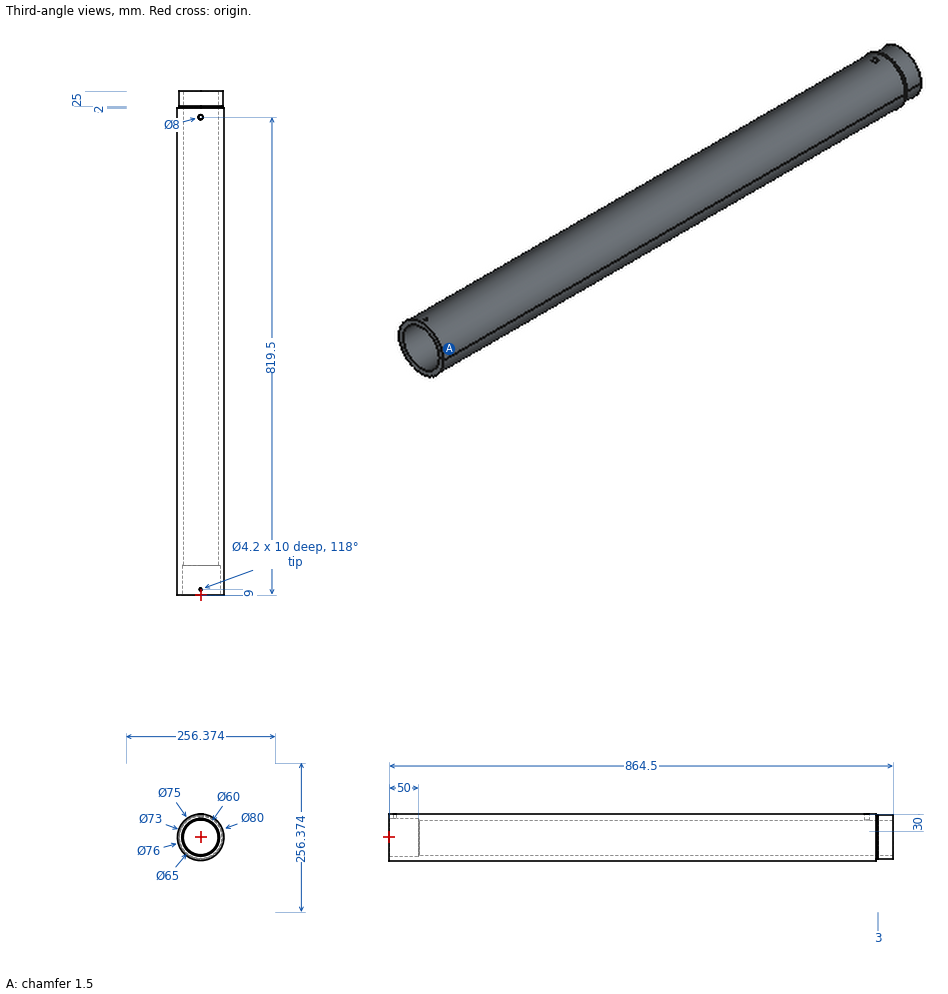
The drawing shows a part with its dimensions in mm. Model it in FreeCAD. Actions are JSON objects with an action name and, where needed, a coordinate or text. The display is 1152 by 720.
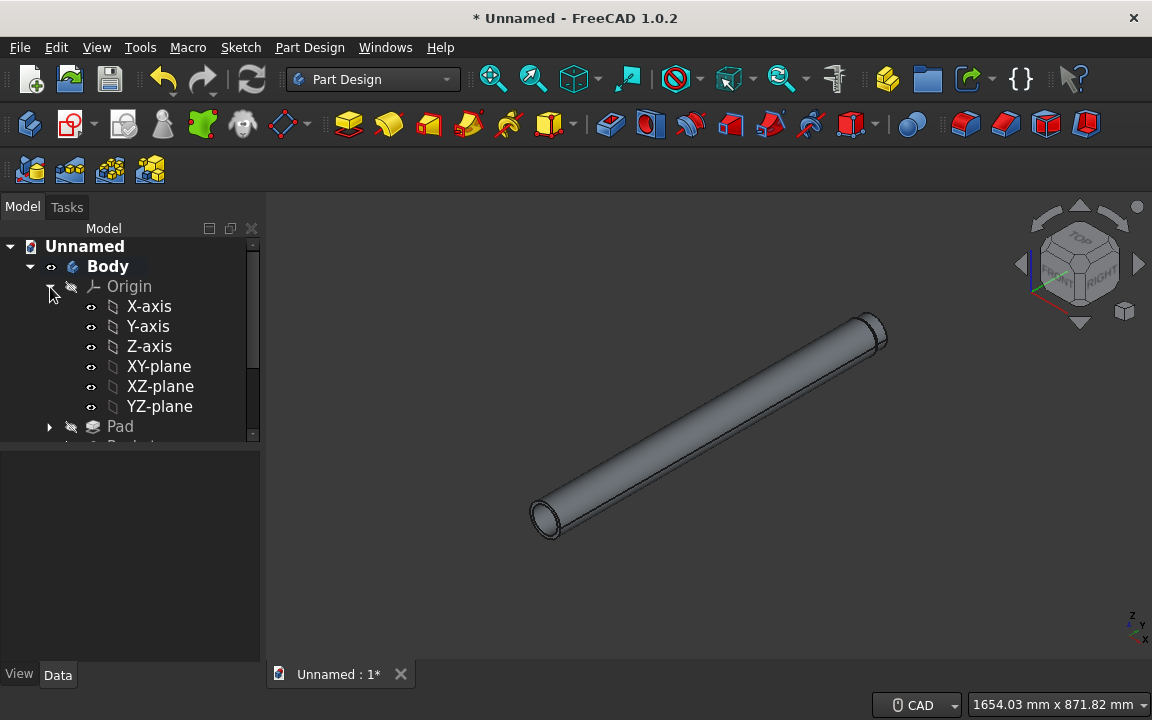
{"action": "left_click", "coordinate": [136, 367]}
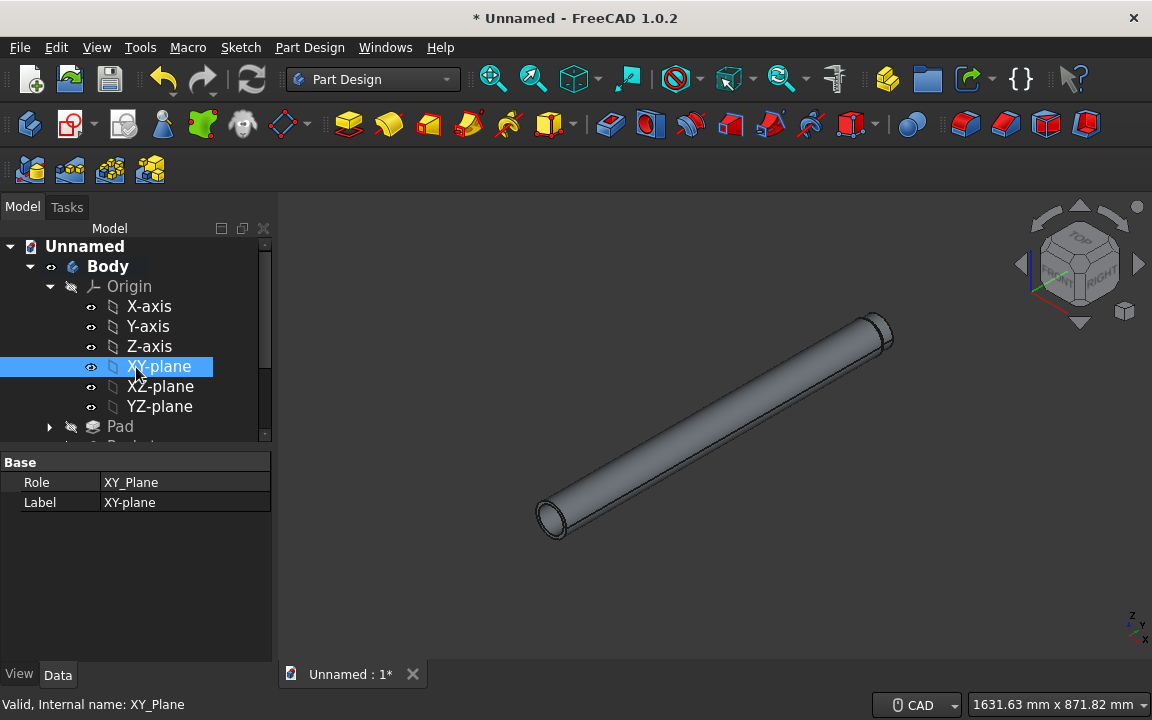
{"action": "left_click", "coordinate": [284, 124]}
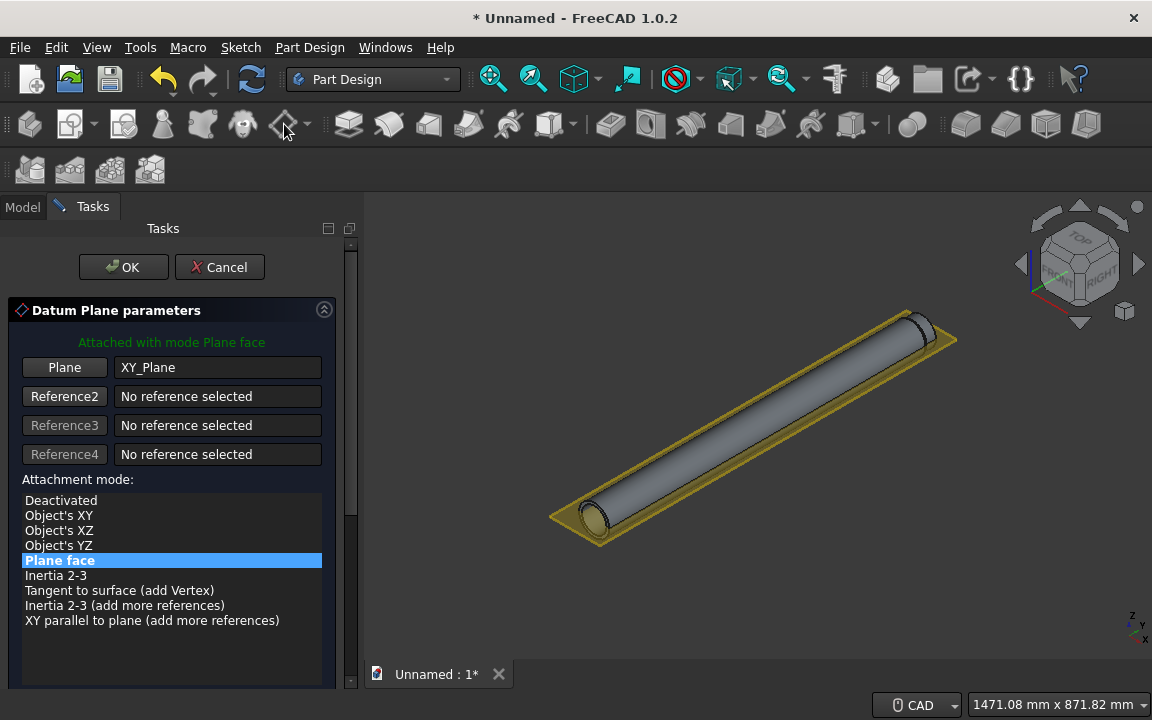
{"action": "scroll", "coordinate": [351, 463], "scroll_direction": "down", "scroll_amount": 3}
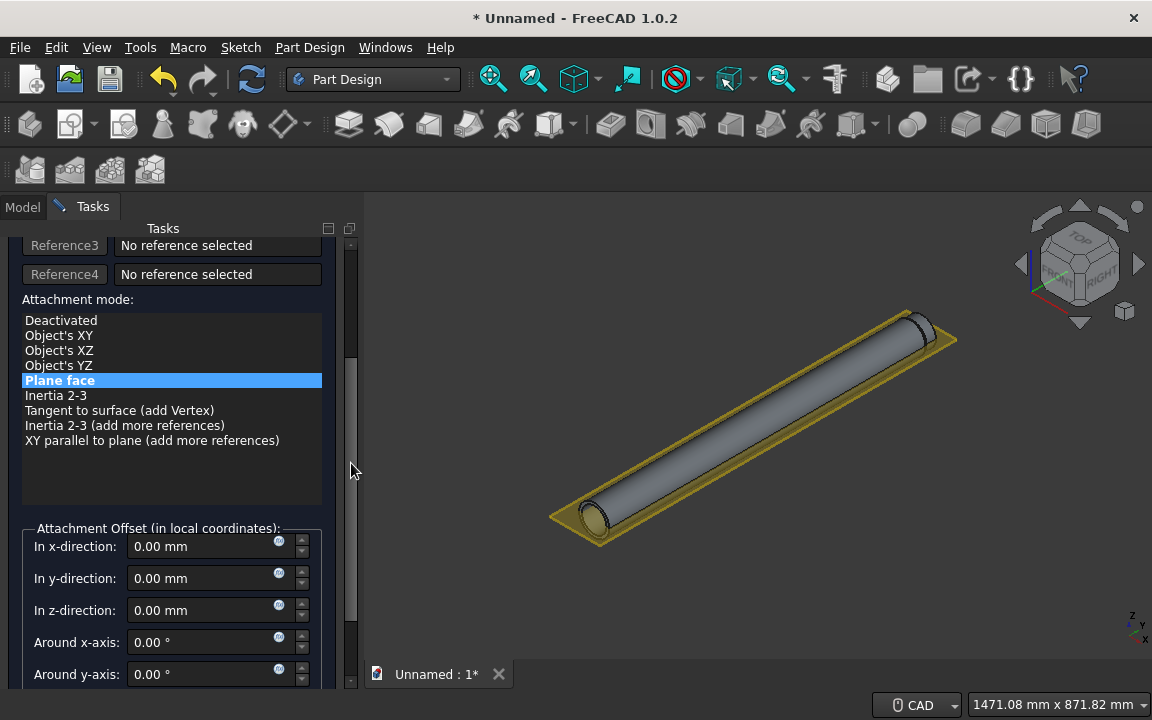
{"action": "triple_click", "coordinate": [210, 610]}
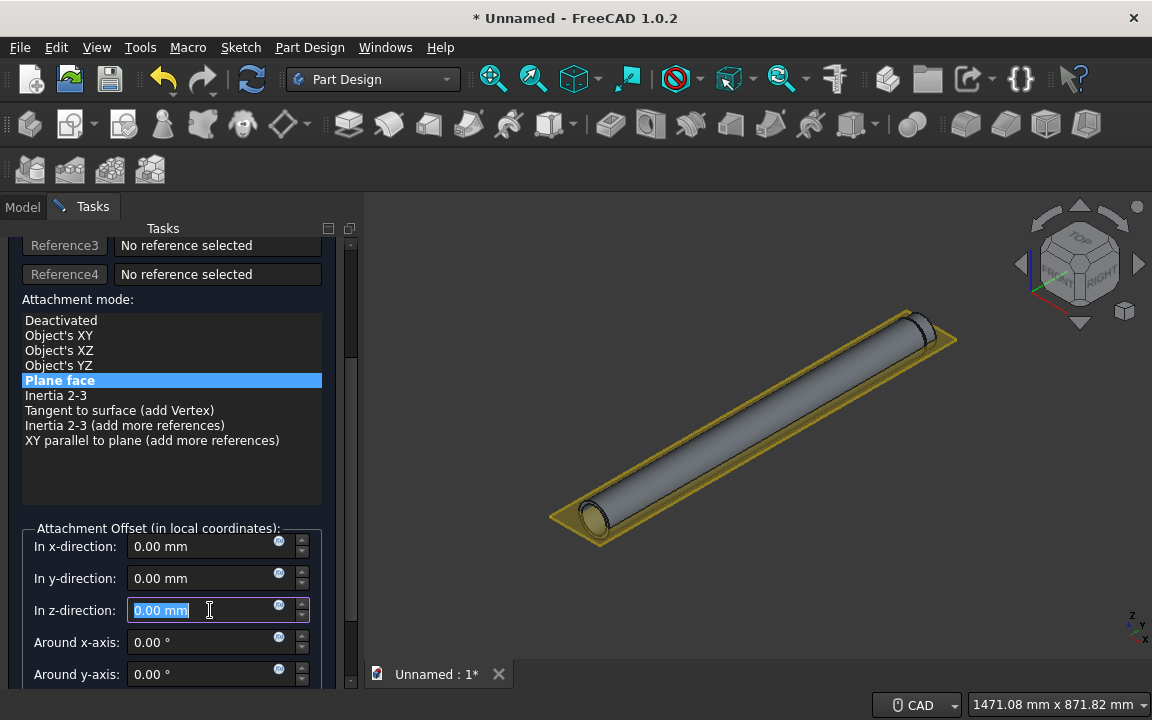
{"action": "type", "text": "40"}
{"action": "key", "text": "Tab"}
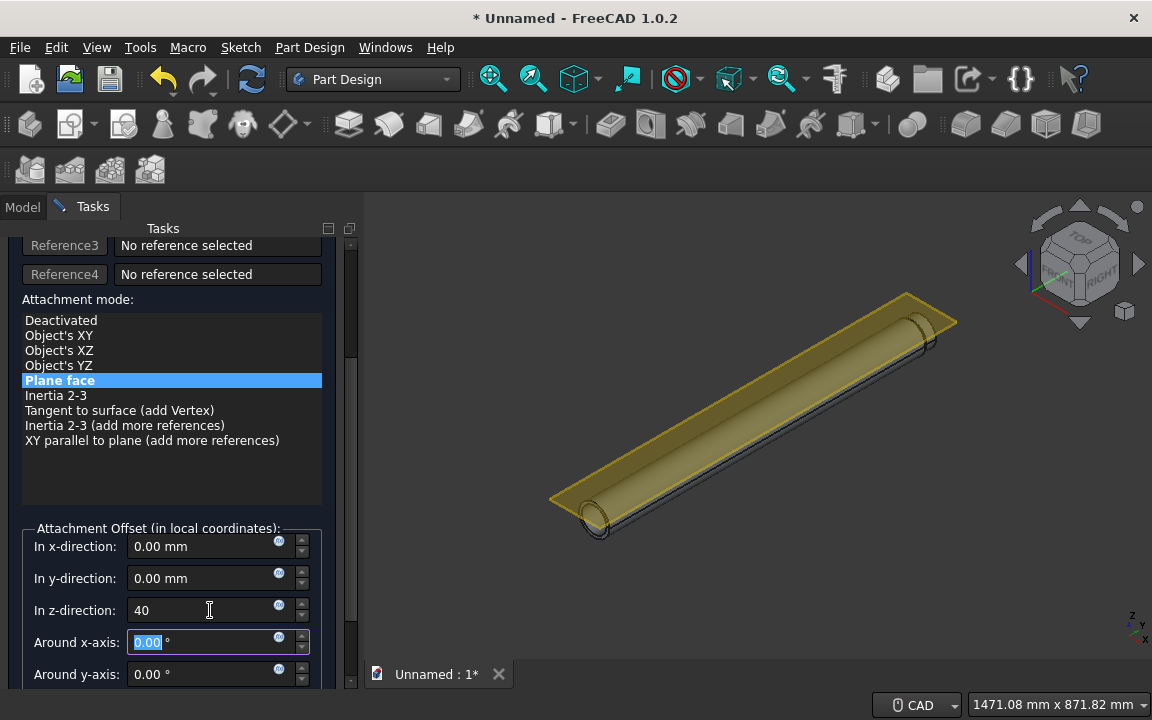
{"action": "scroll", "coordinate": [351, 463], "scroll_direction": "up", "scroll_amount": 4}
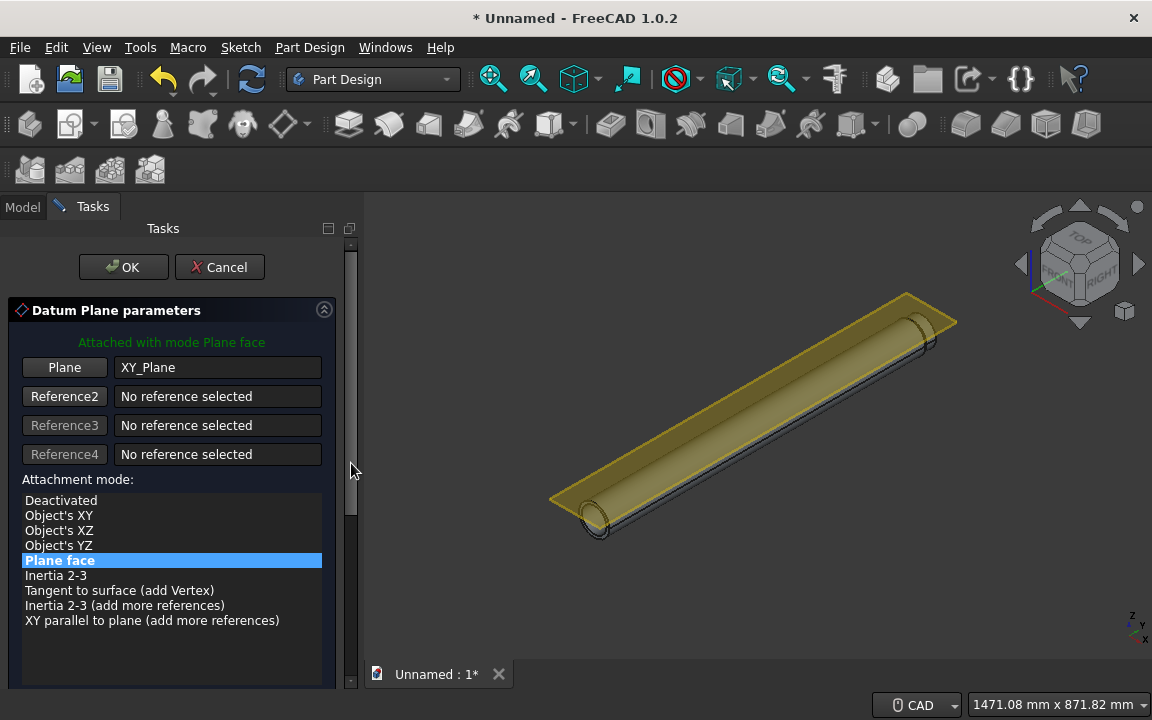
{"action": "left_click", "coordinate": [124, 267]}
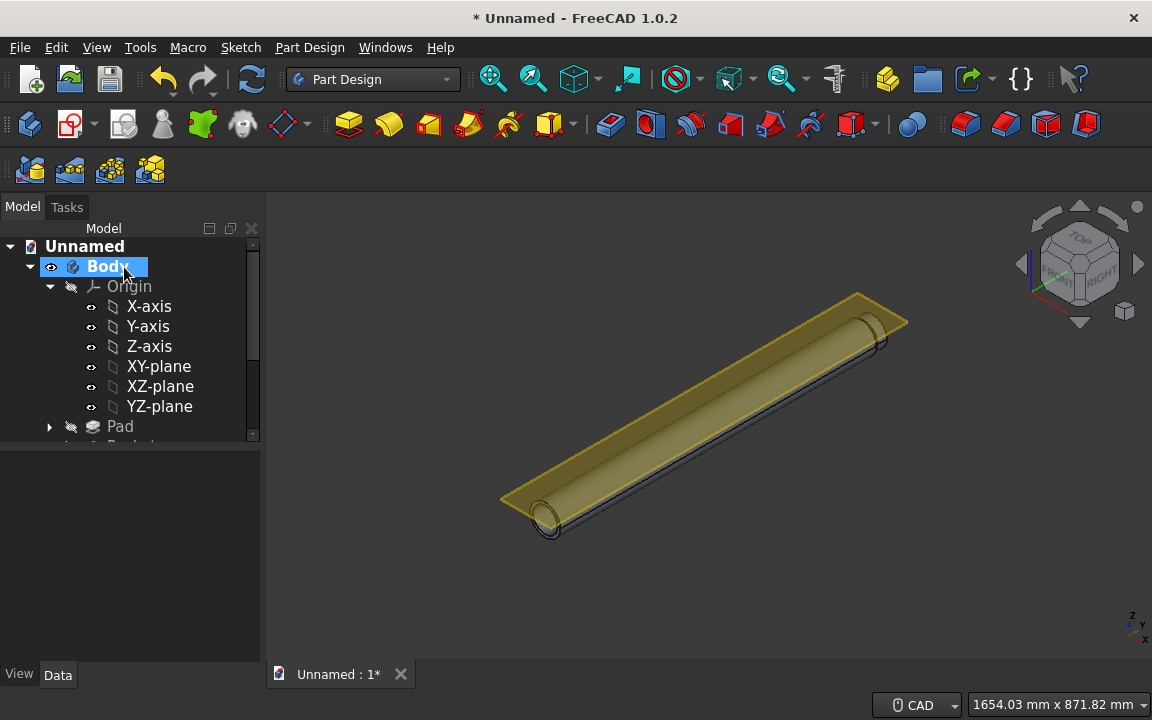
{"action": "scroll", "coordinate": [100, 342], "scroll_direction": "down", "scroll_amount": 3}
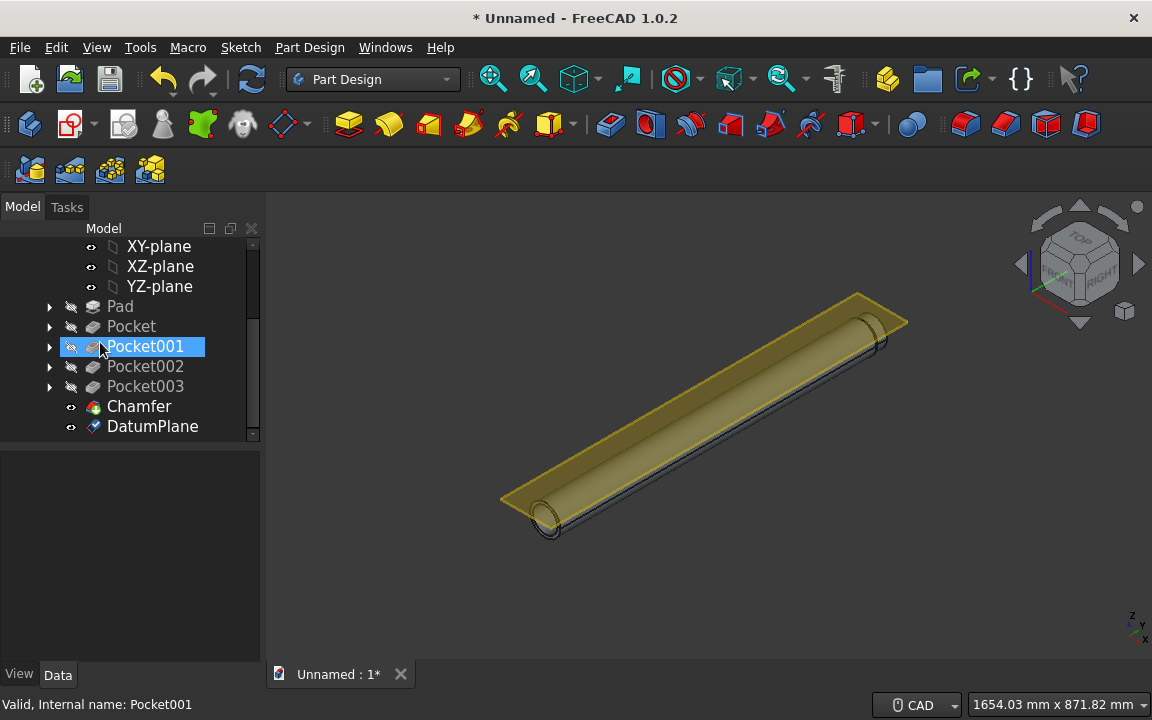
{"action": "left_click", "coordinate": [116, 427]}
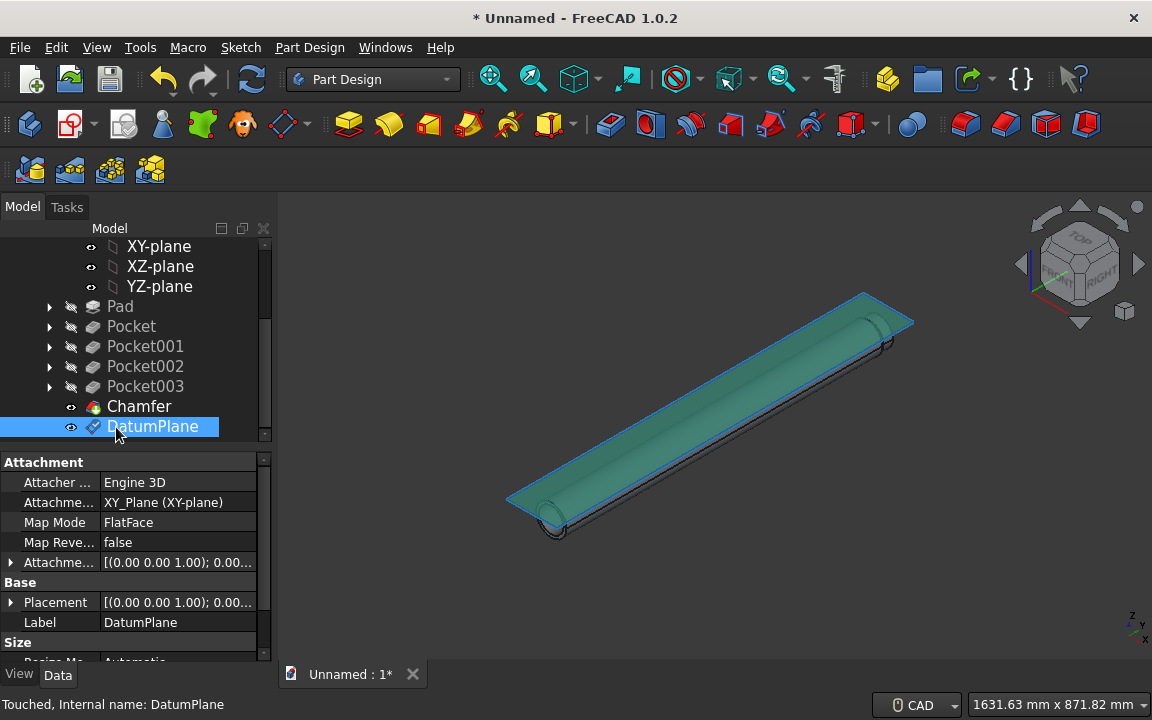
{"action": "left_click", "coordinate": [70, 124]}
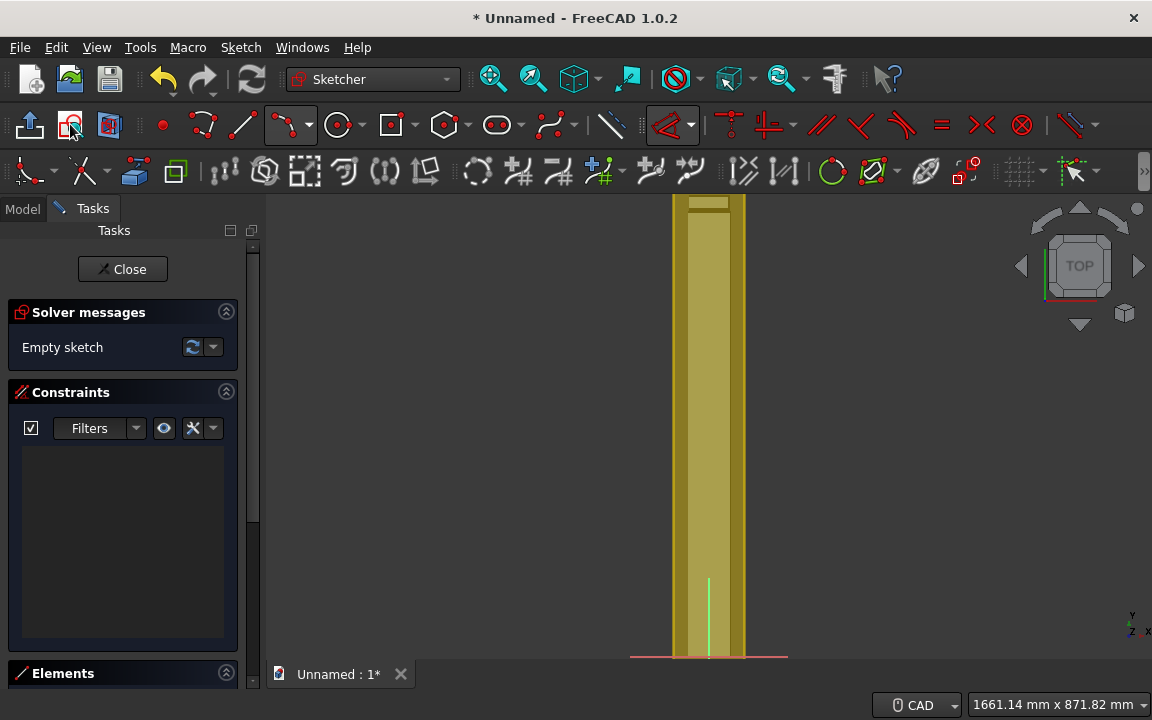
{"action": "scroll", "coordinate": [640, 426], "scroll_direction": "down", "scroll_amount": 5}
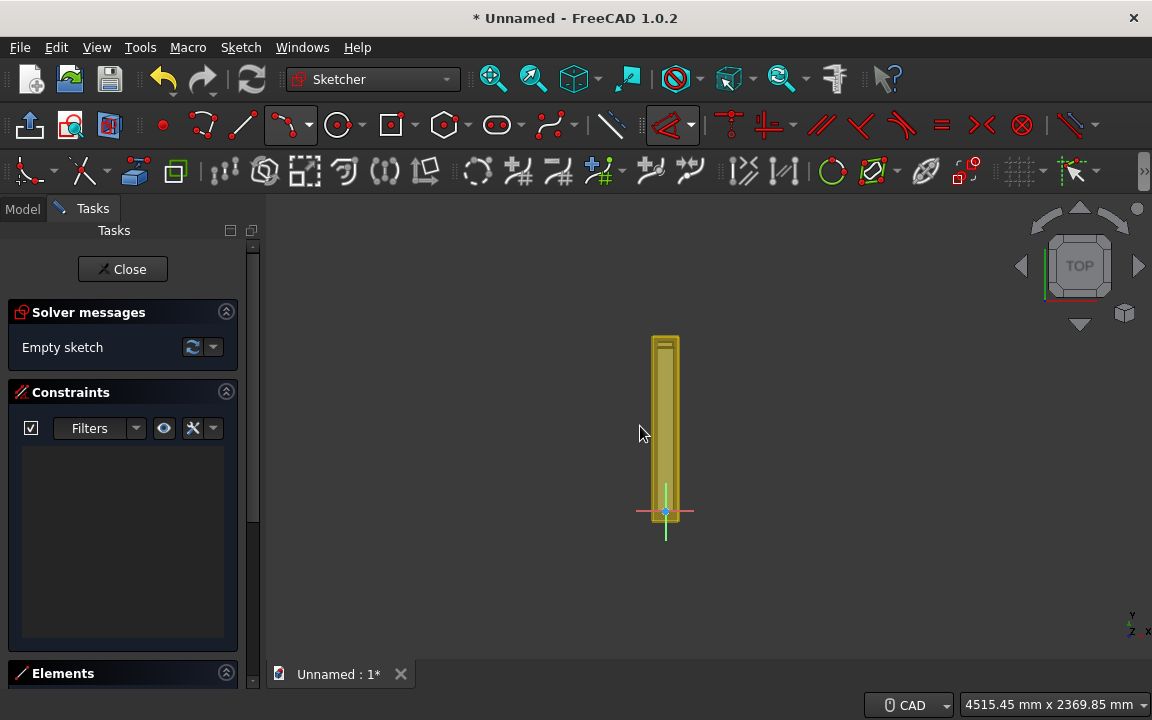
{"action": "scroll", "coordinate": [667, 514], "scroll_direction": "up", "scroll_amount": 15}